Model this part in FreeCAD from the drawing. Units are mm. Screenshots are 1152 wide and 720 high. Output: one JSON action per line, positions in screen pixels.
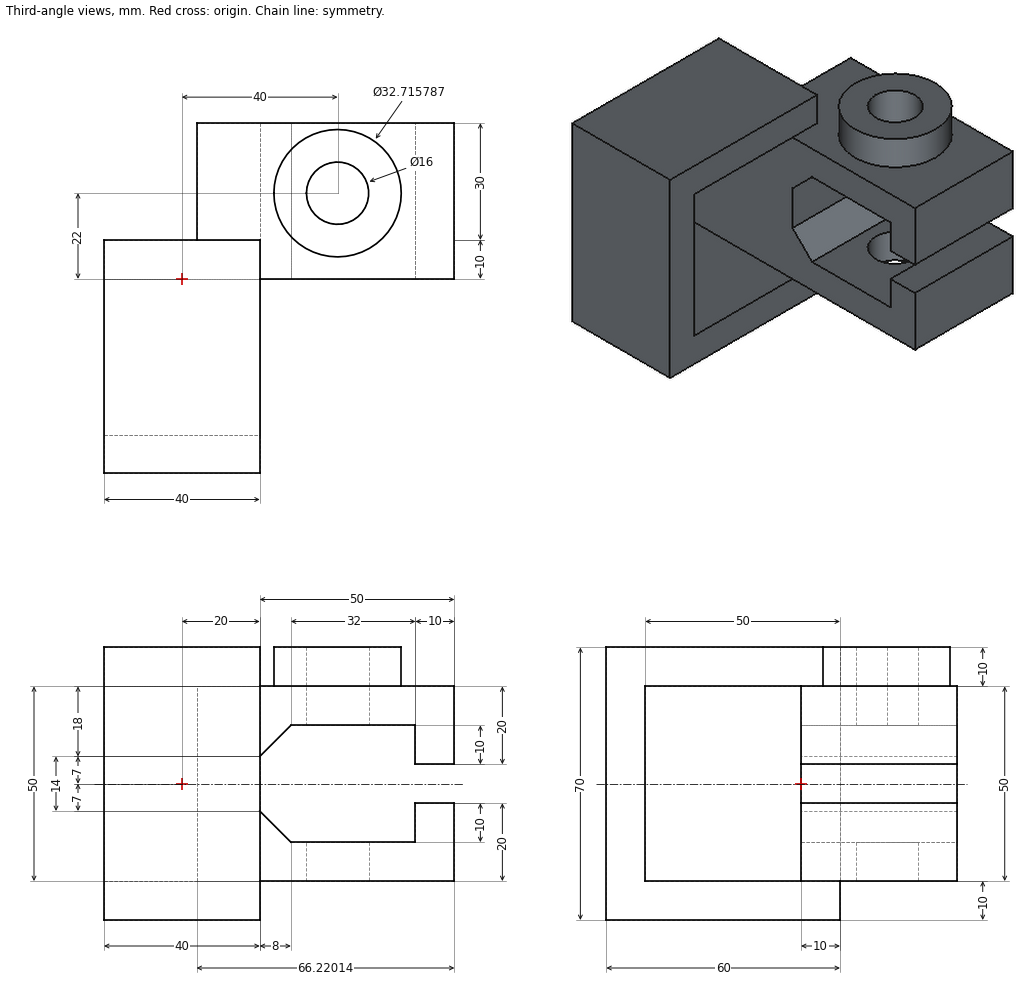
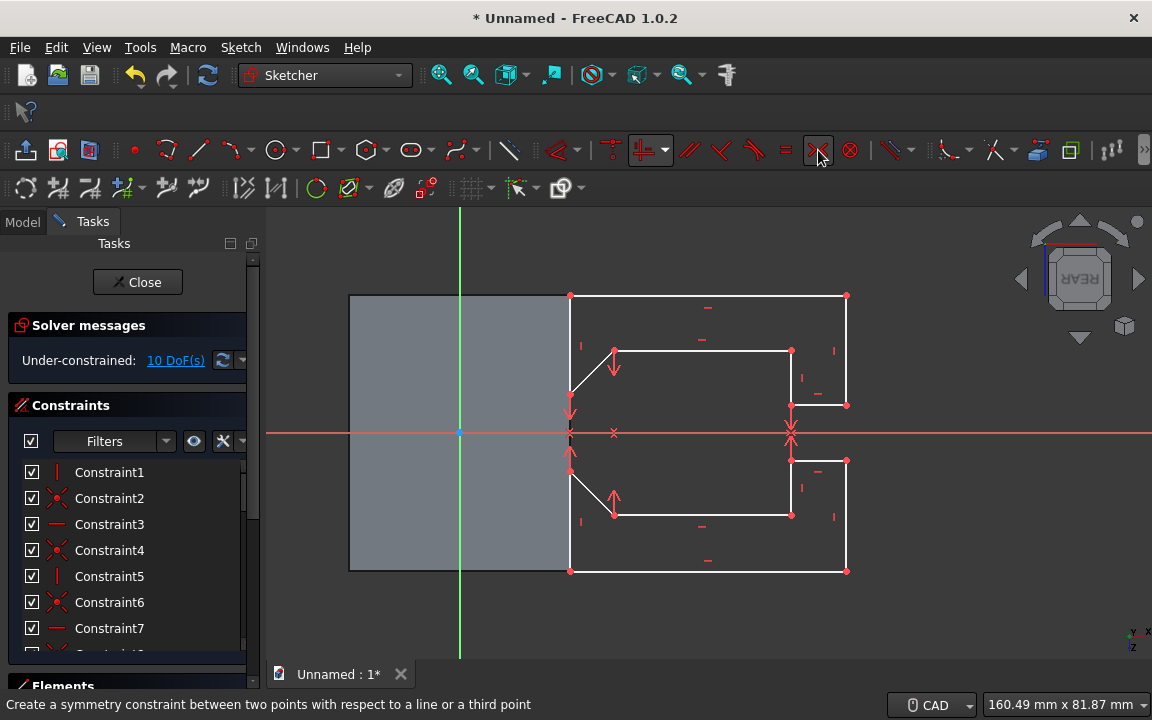
{"action": "left_click", "coordinate": [846, 572]}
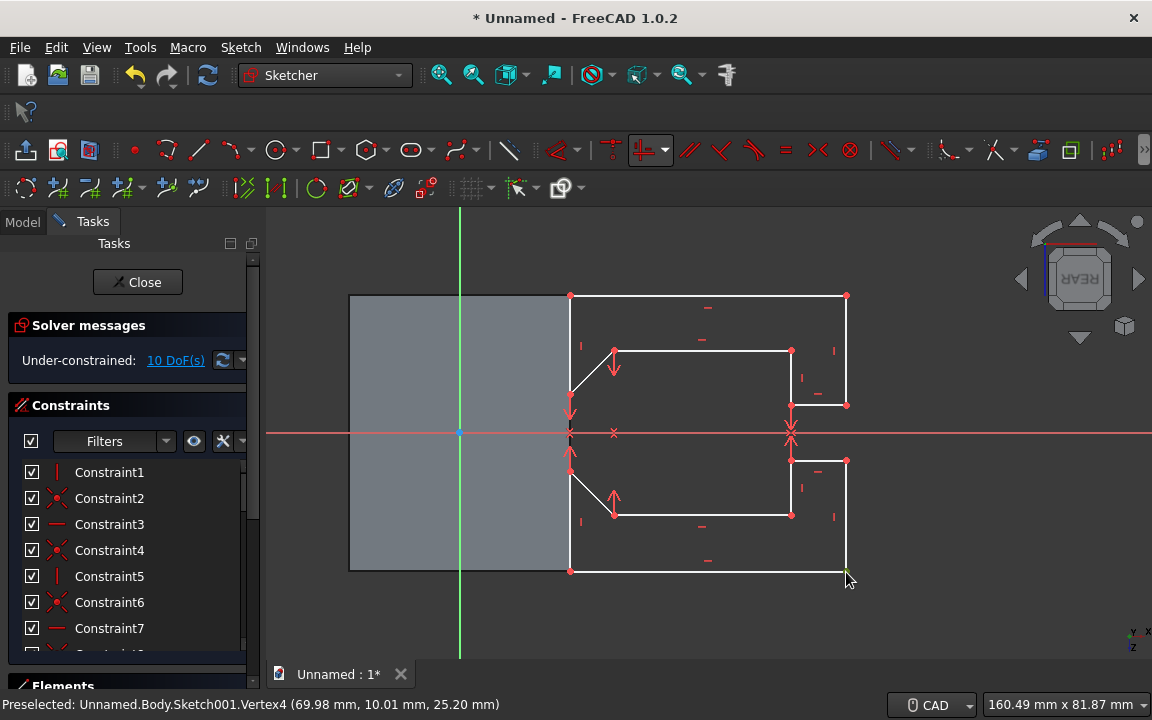
{"action": "left_click", "coordinate": [846, 296]}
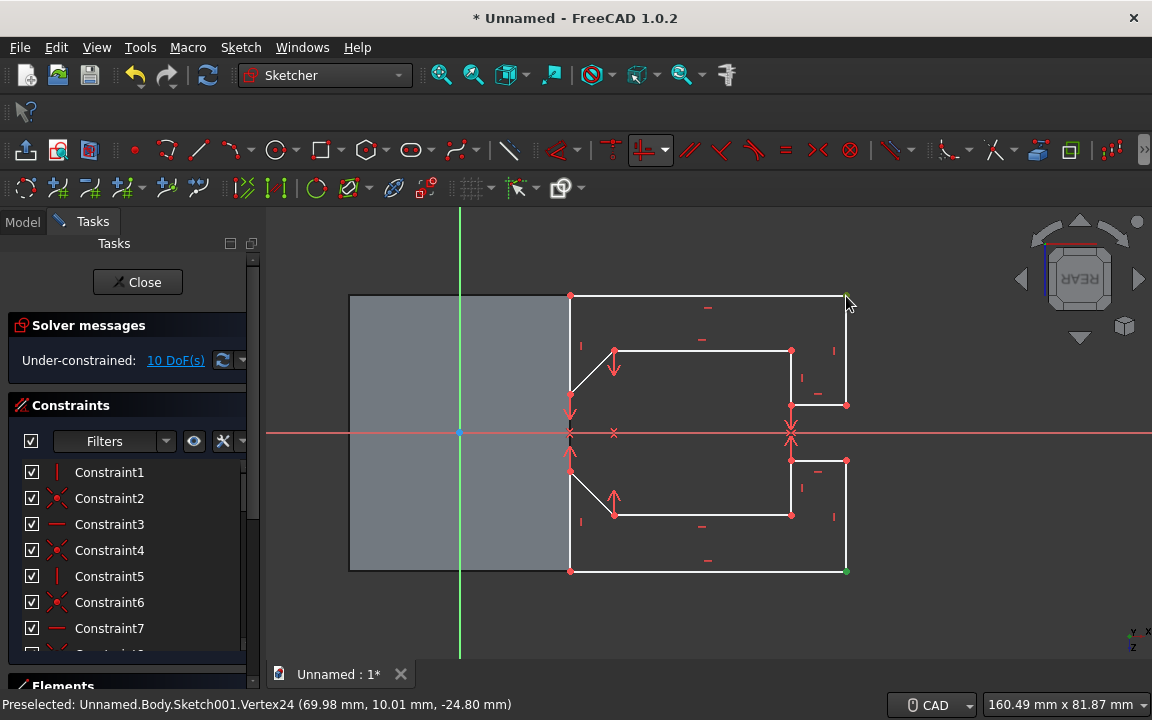
{"action": "left_click", "coordinate": [344, 433]}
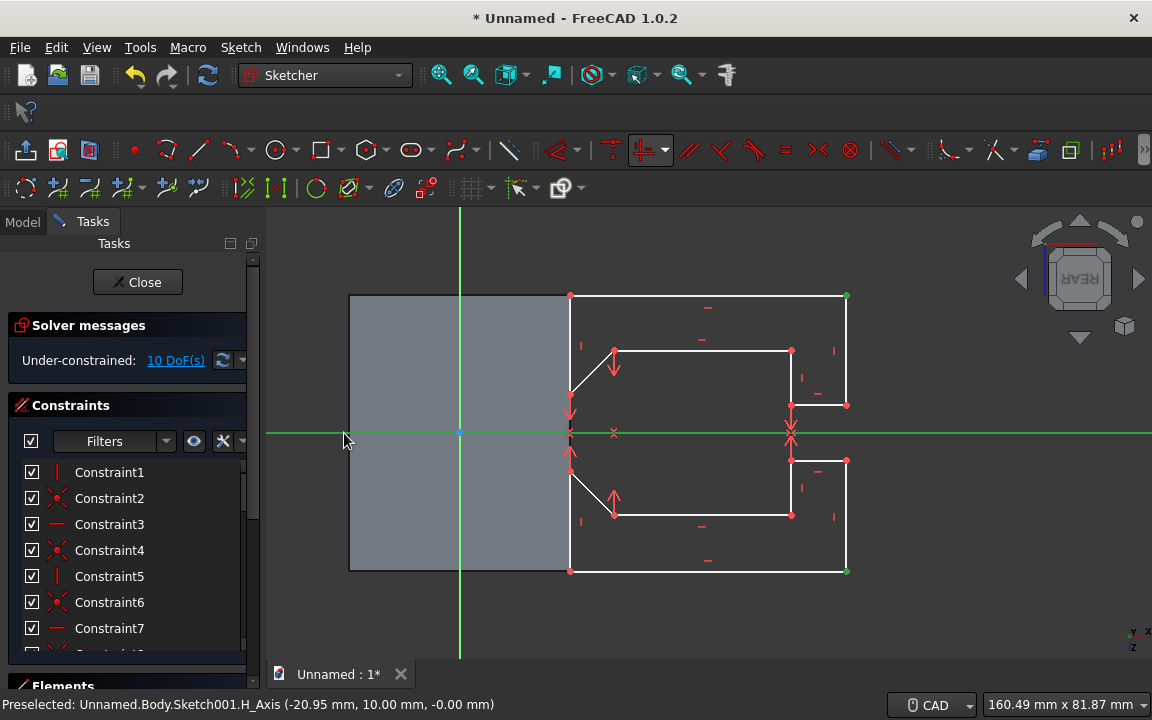
{"action": "key", "text": "s"}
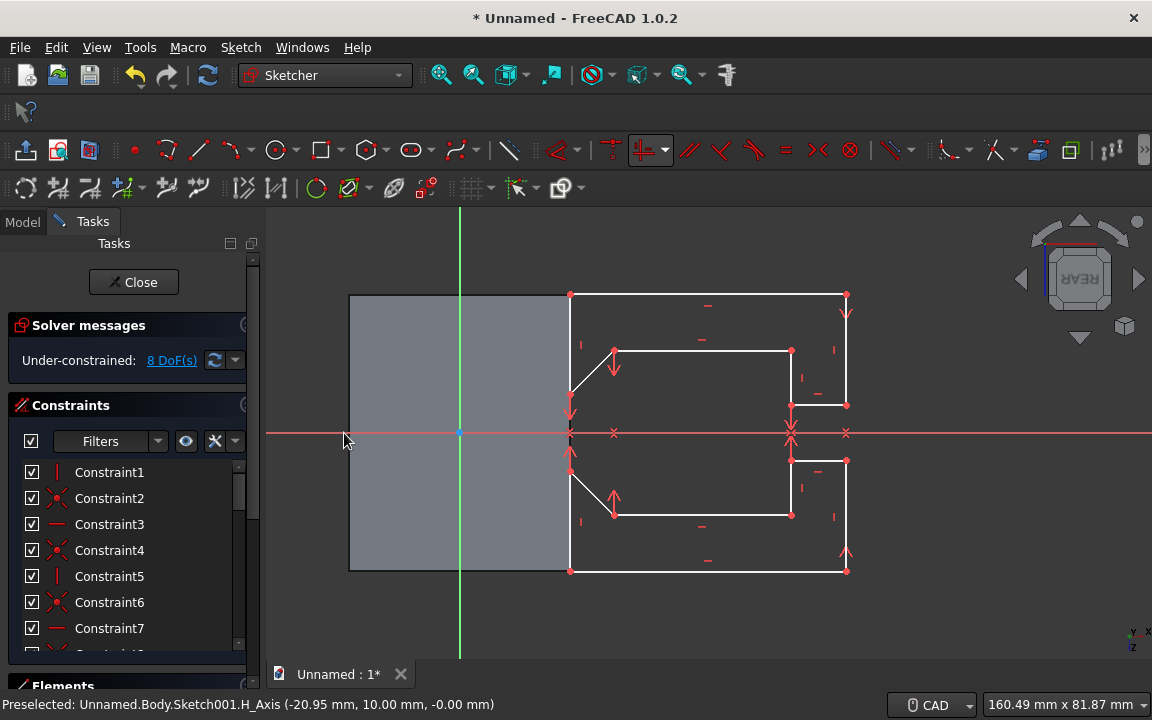
{"action": "key", "text": "d"}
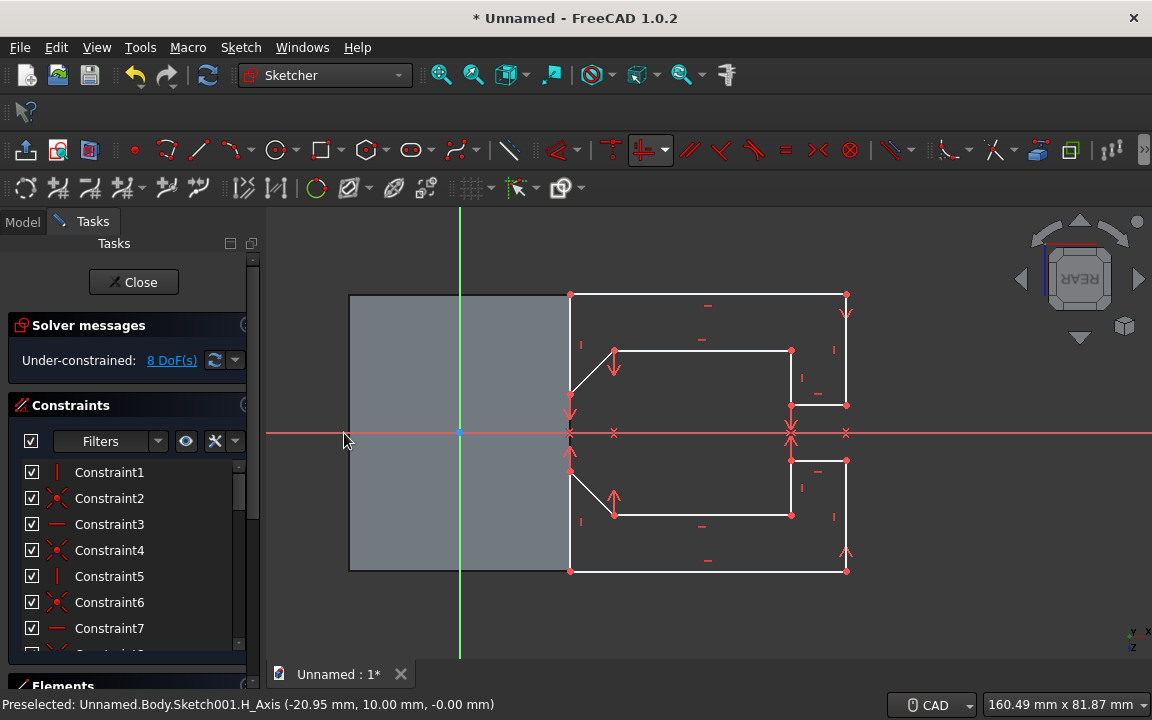
{"action": "left_click", "coordinate": [570, 501]}
{"action": "left_click", "coordinate": [536, 521]}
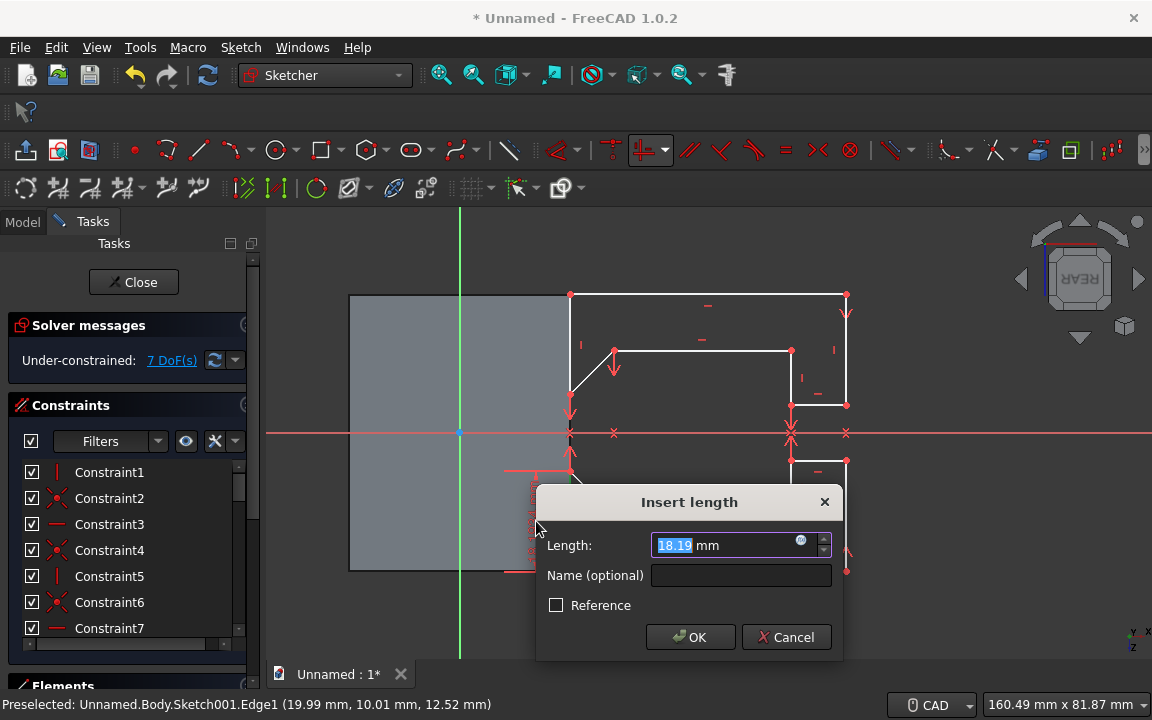
{"action": "type", "text": "18"}
{"action": "key", "text": "Return"}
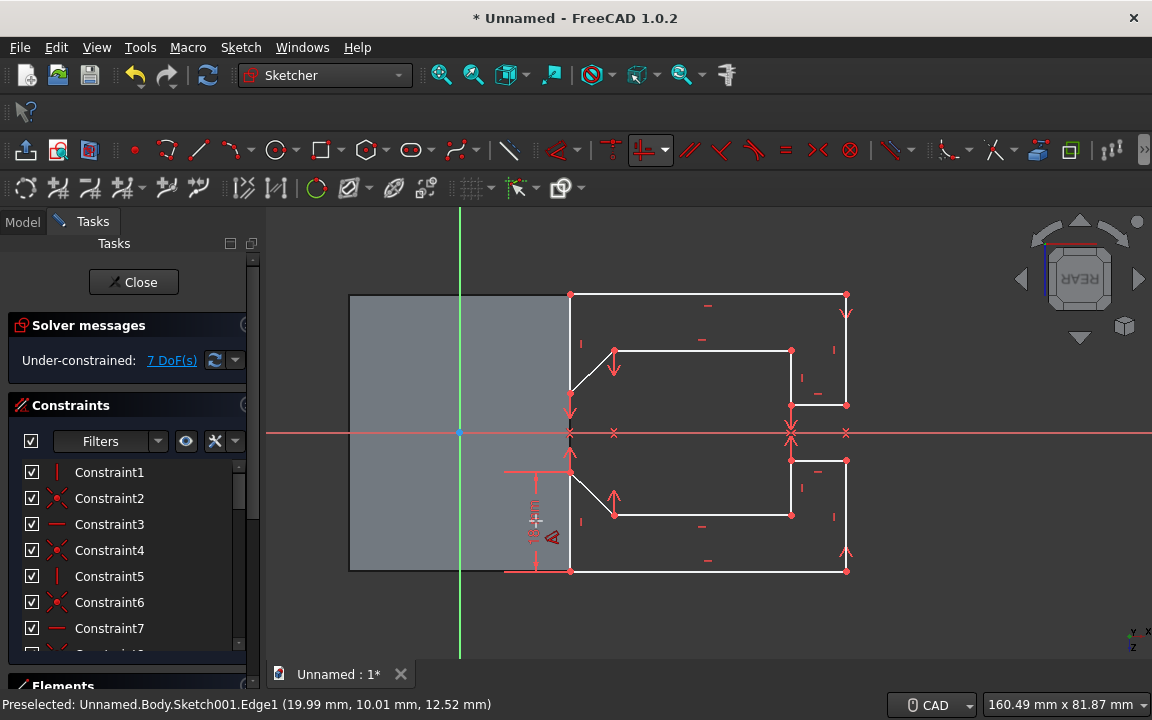
{"action": "left_click", "coordinate": [653, 572]}
{"action": "left_click", "coordinate": [708, 606]}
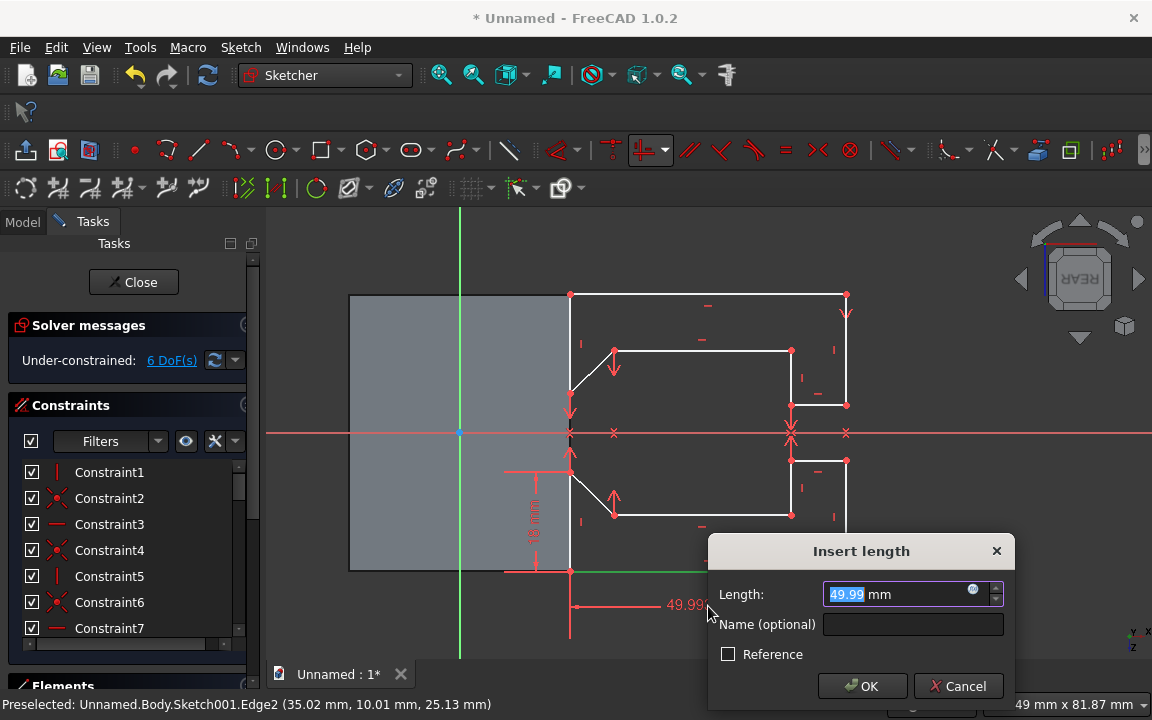
{"action": "type", "text": "50"}
{"action": "key", "text": "Return"}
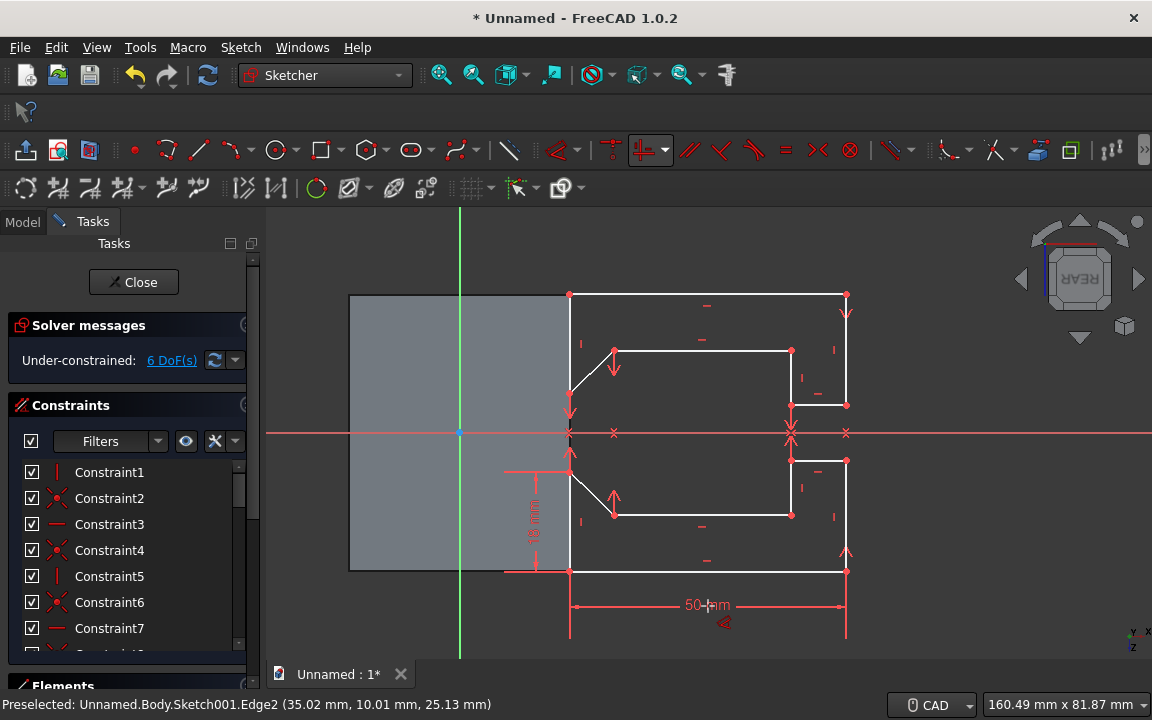
{"action": "left_click", "coordinate": [846, 538]}
{"action": "left_click", "coordinate": [880, 516]}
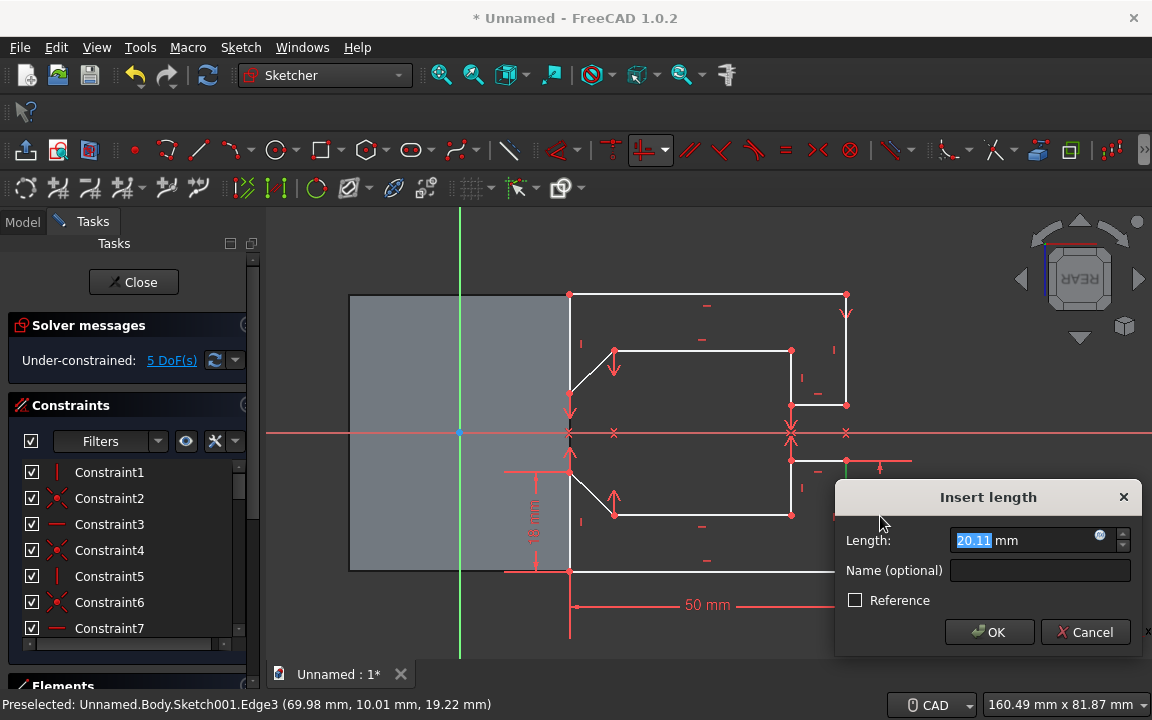
{"action": "type", "text": "20"}
{"action": "key", "text": "Return"}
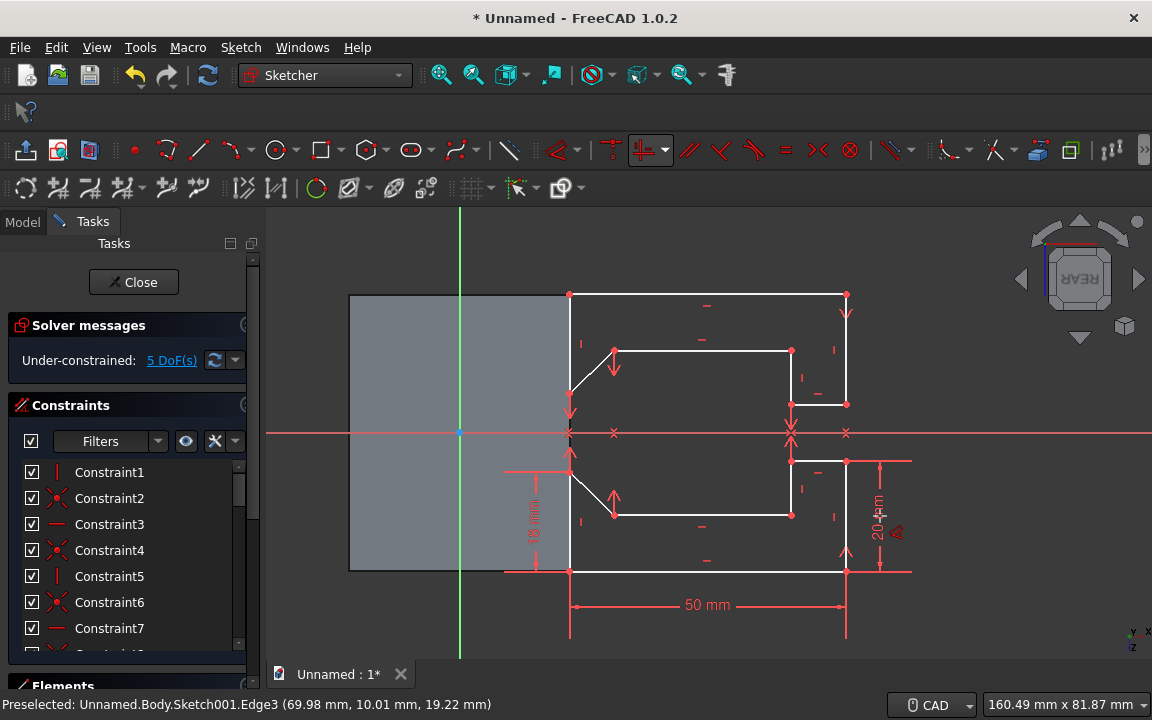
{"action": "left_click", "coordinate": [830, 461]}
{"action": "left_click", "coordinate": [819, 495]}